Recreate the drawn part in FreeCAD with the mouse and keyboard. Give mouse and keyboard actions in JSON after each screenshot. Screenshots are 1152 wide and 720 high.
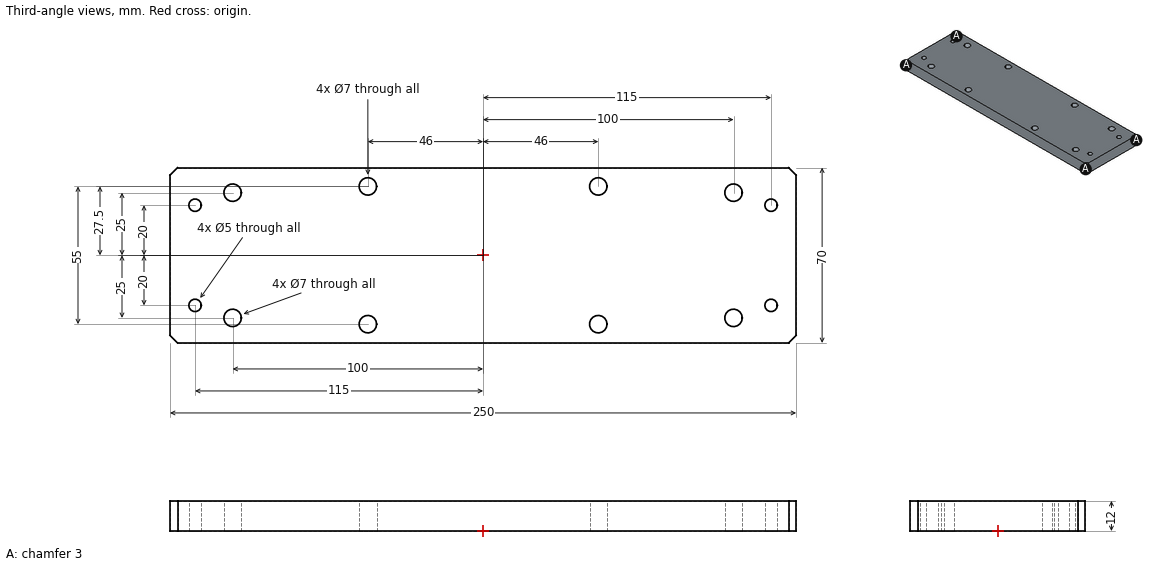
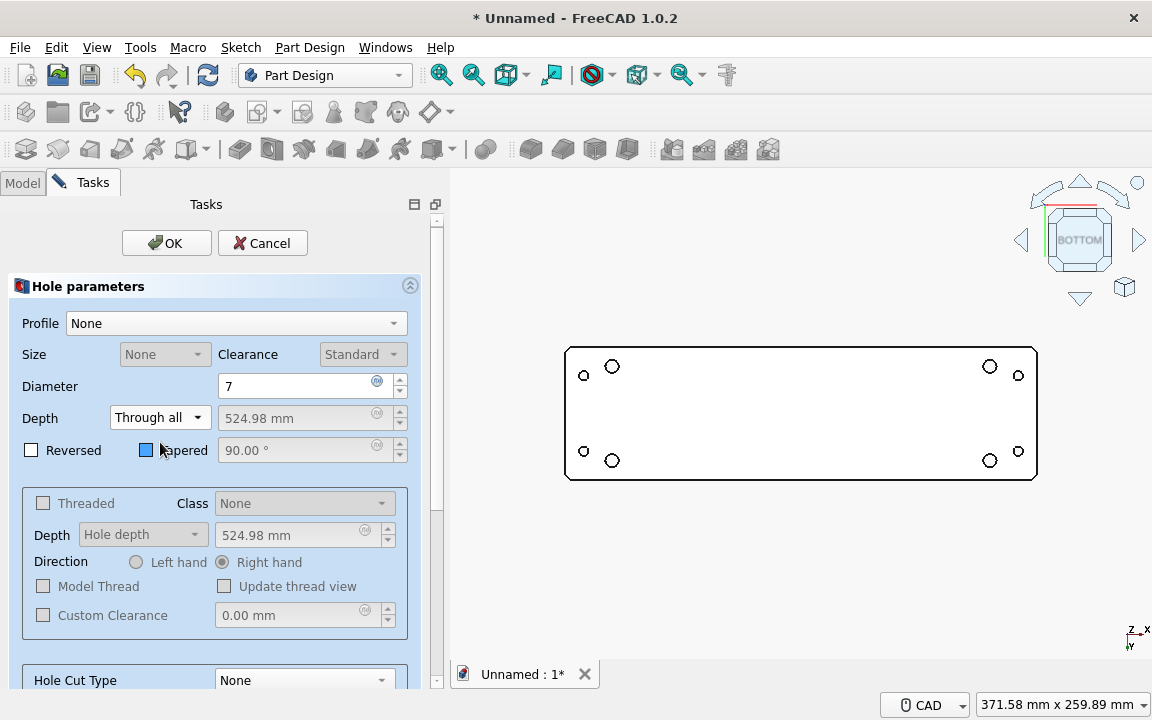
{"action": "left_click", "coordinate": [30, 450]}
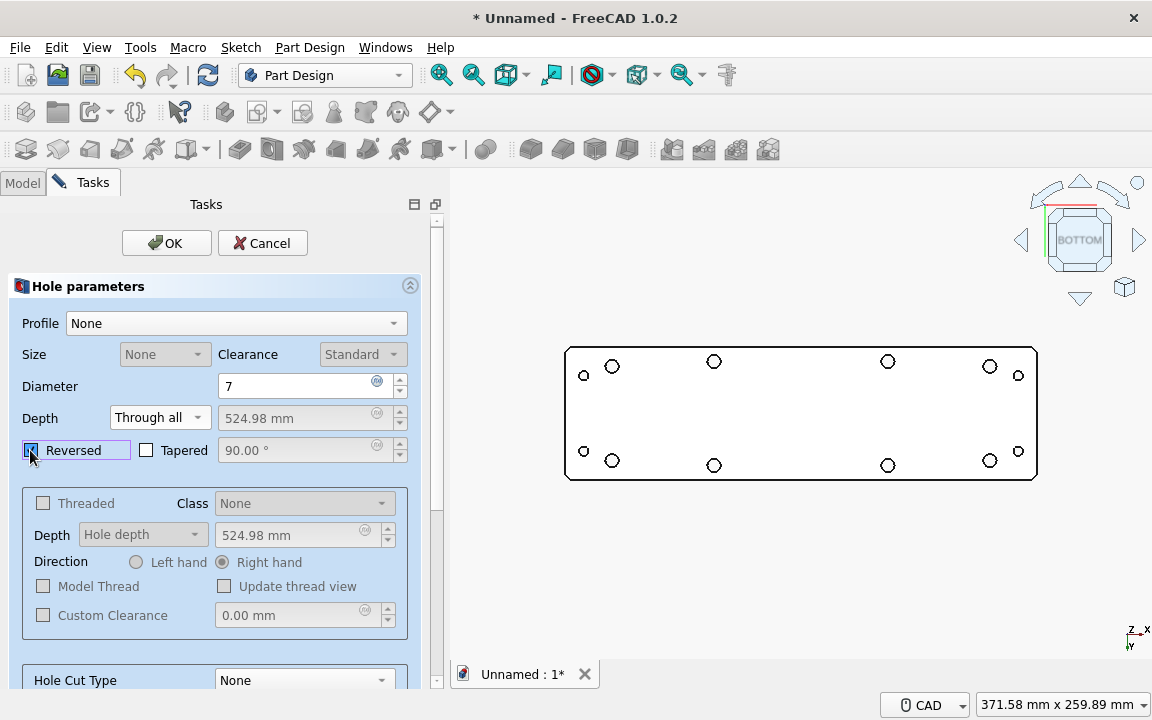
{"action": "left_click", "coordinate": [167, 243]}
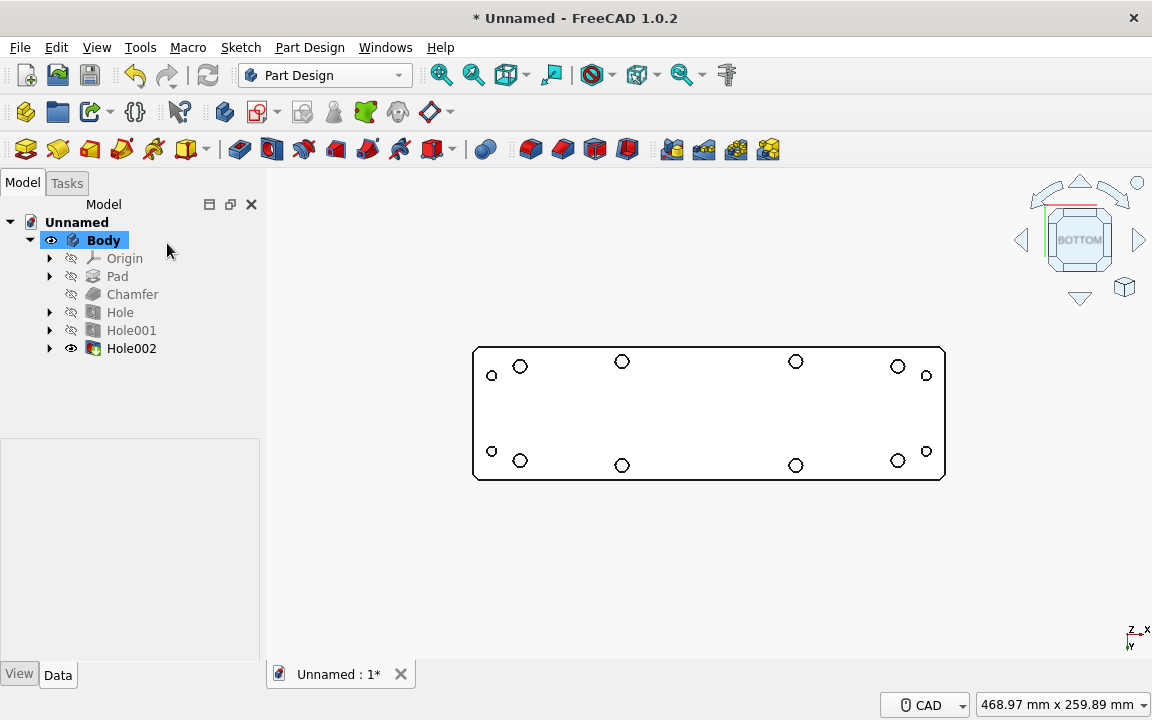
{"action": "key", "text": "0"}